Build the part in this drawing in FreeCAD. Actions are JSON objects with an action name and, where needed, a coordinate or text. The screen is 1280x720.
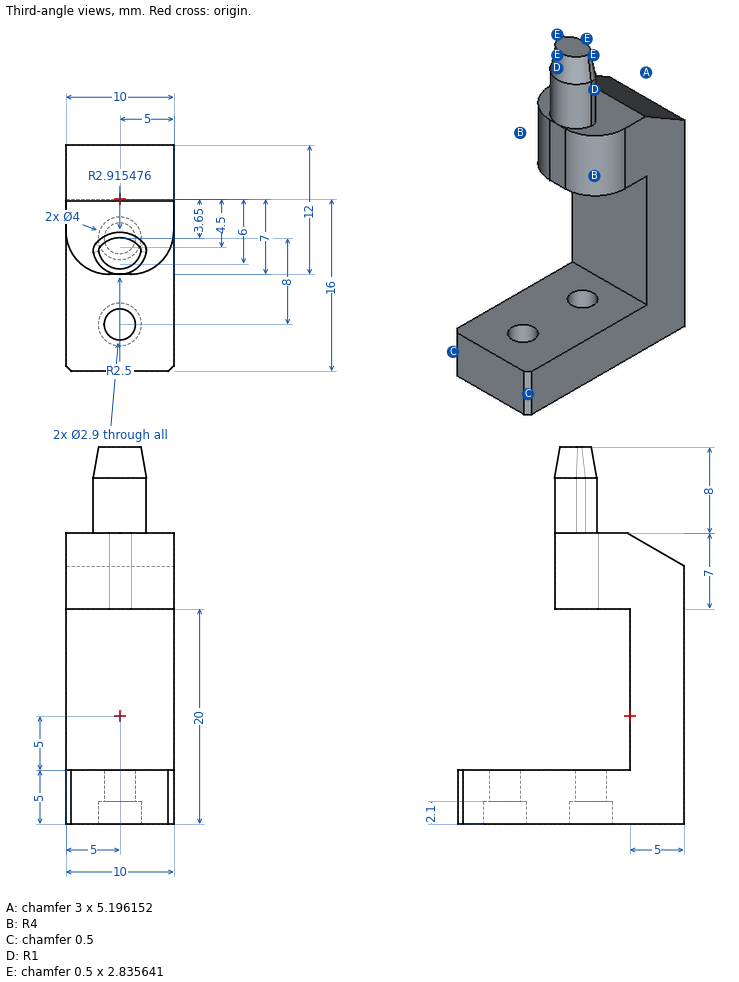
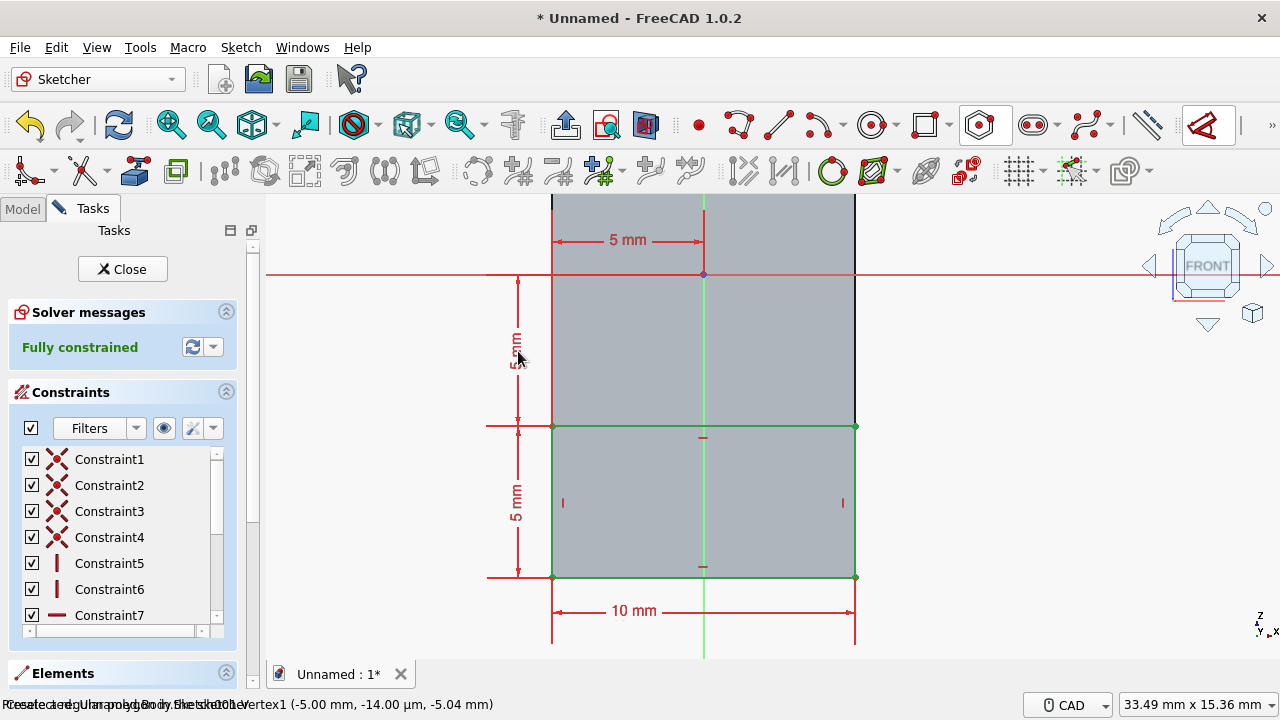
{"action": "left_click", "coordinate": [123, 269]}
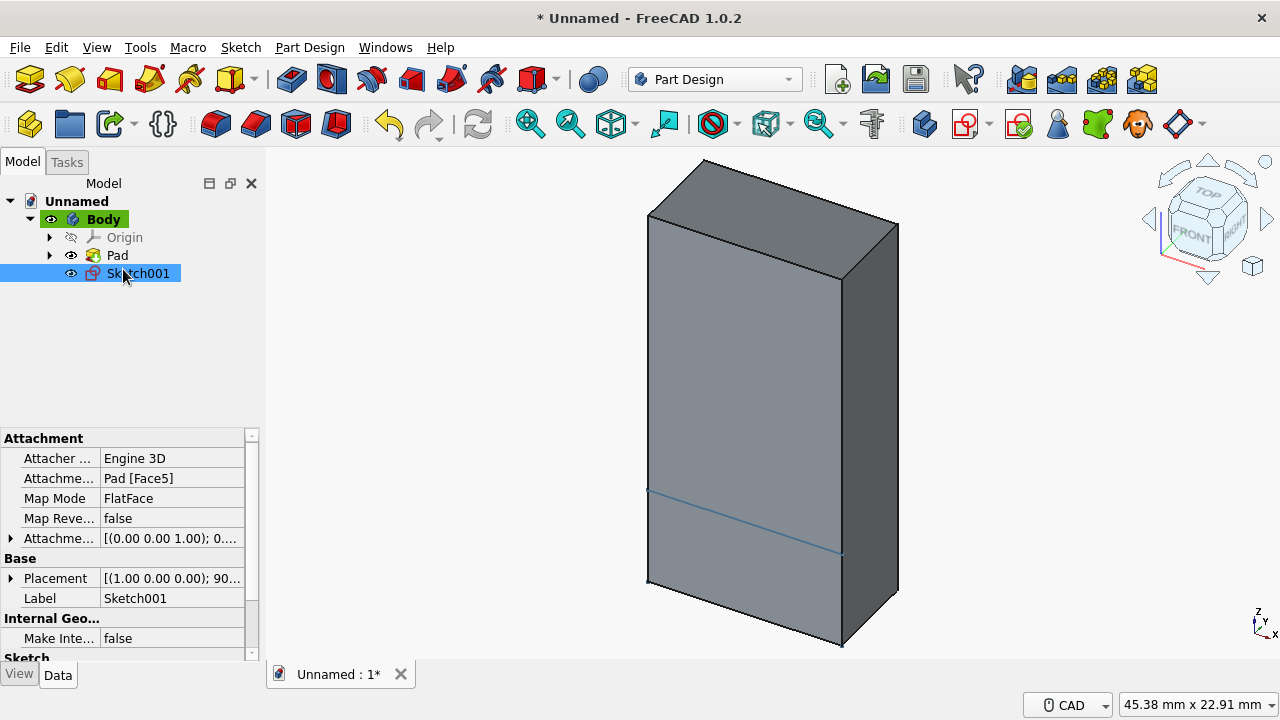
{"action": "left_click", "coordinate": [30, 80]}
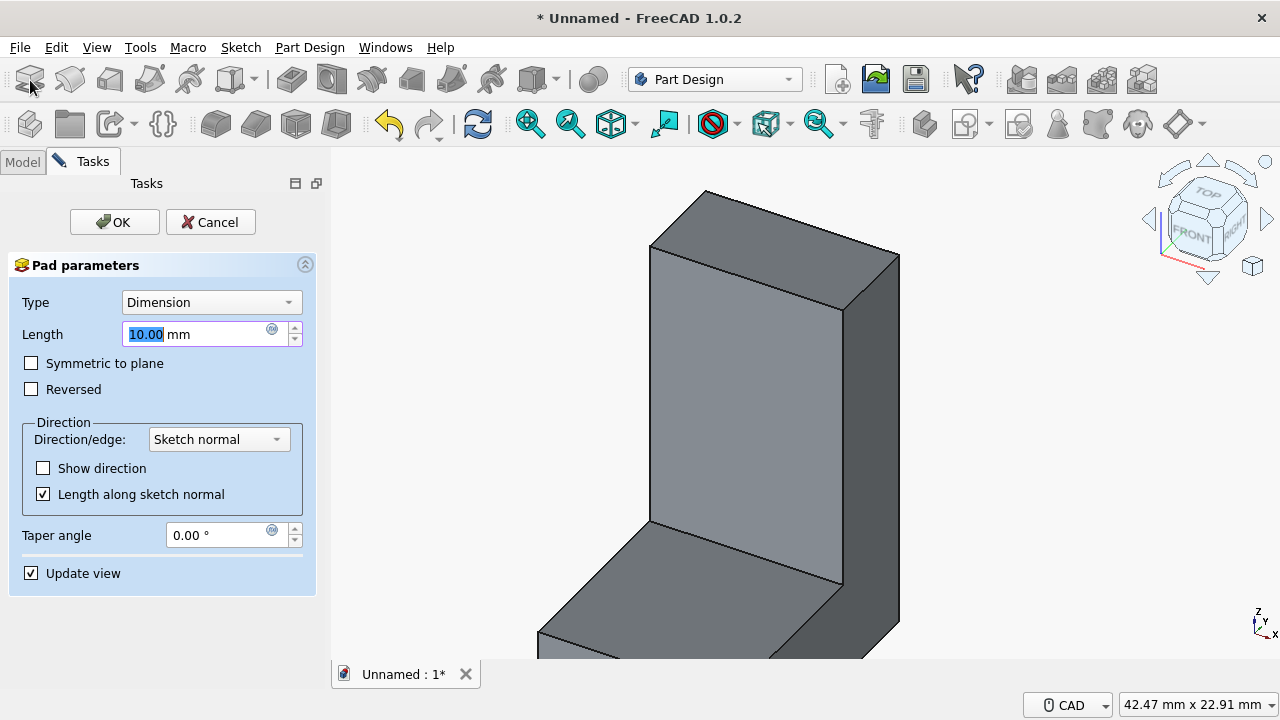
{"action": "type", "text": "16"}
{"action": "key", "text": "Tab"}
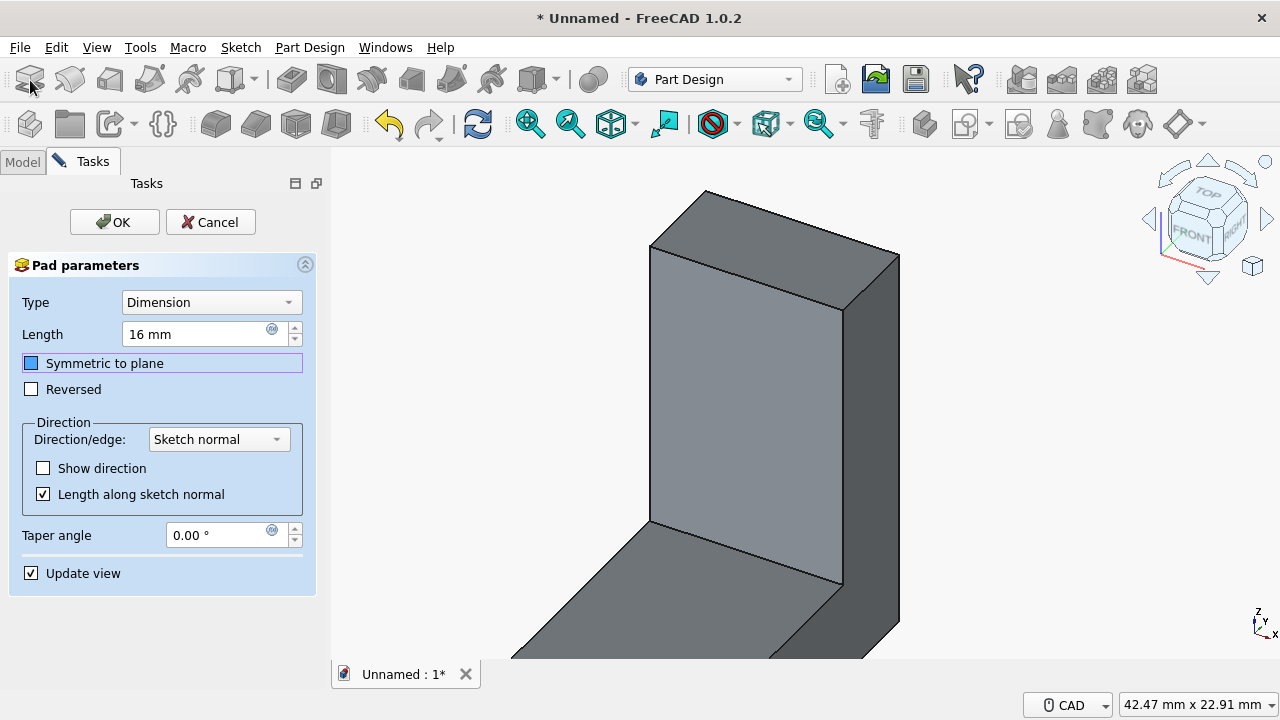
{"action": "left_click", "coordinate": [115, 222]}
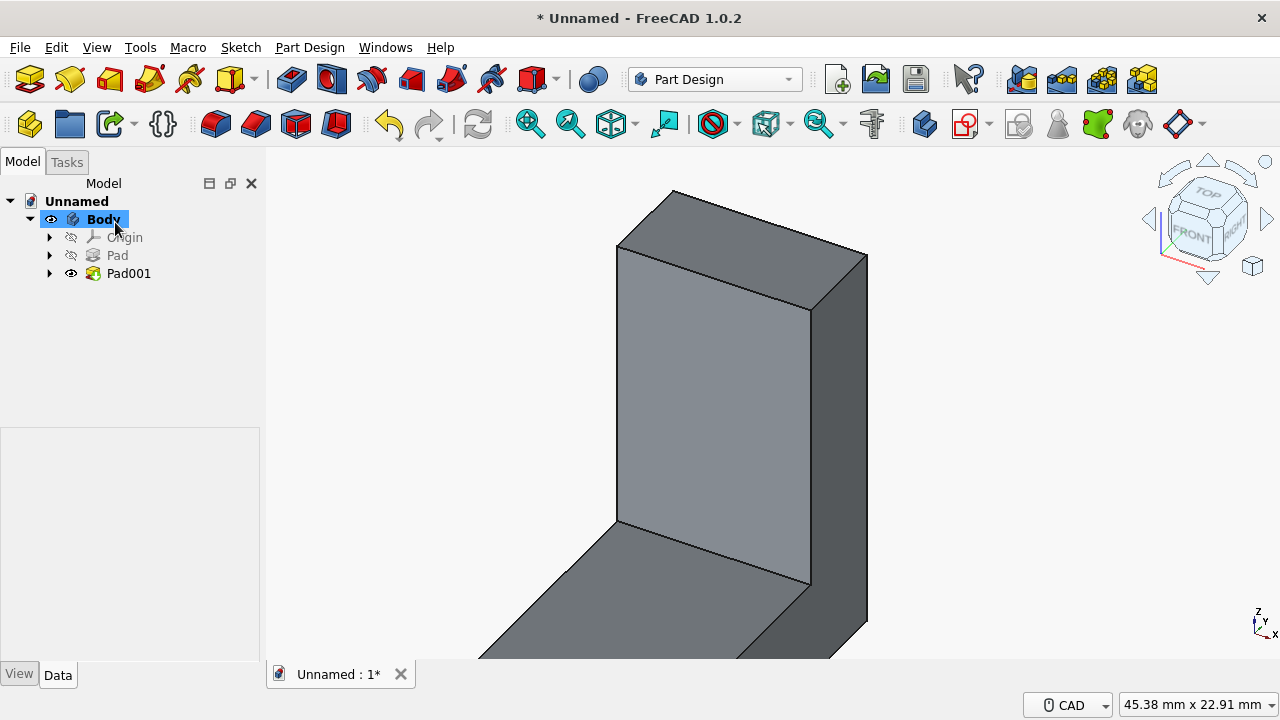
{"action": "left_click", "coordinate": [532, 124]}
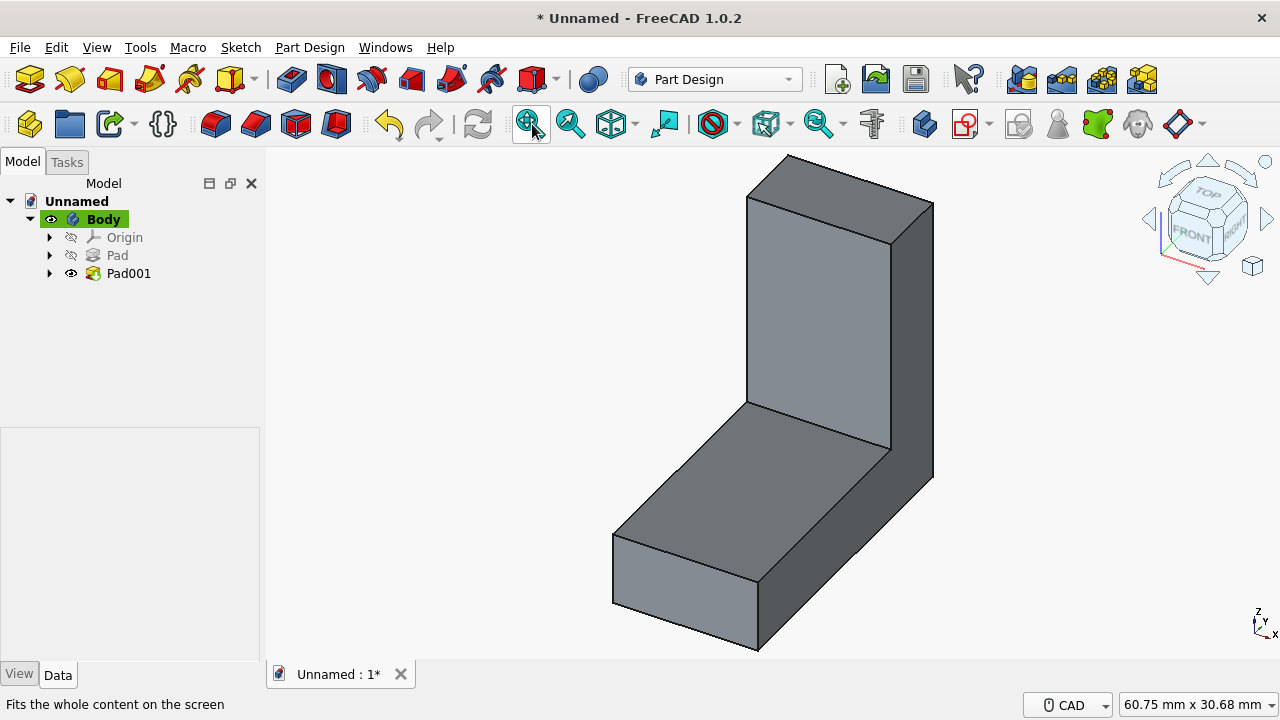
{"action": "left_click", "coordinate": [771, 472]}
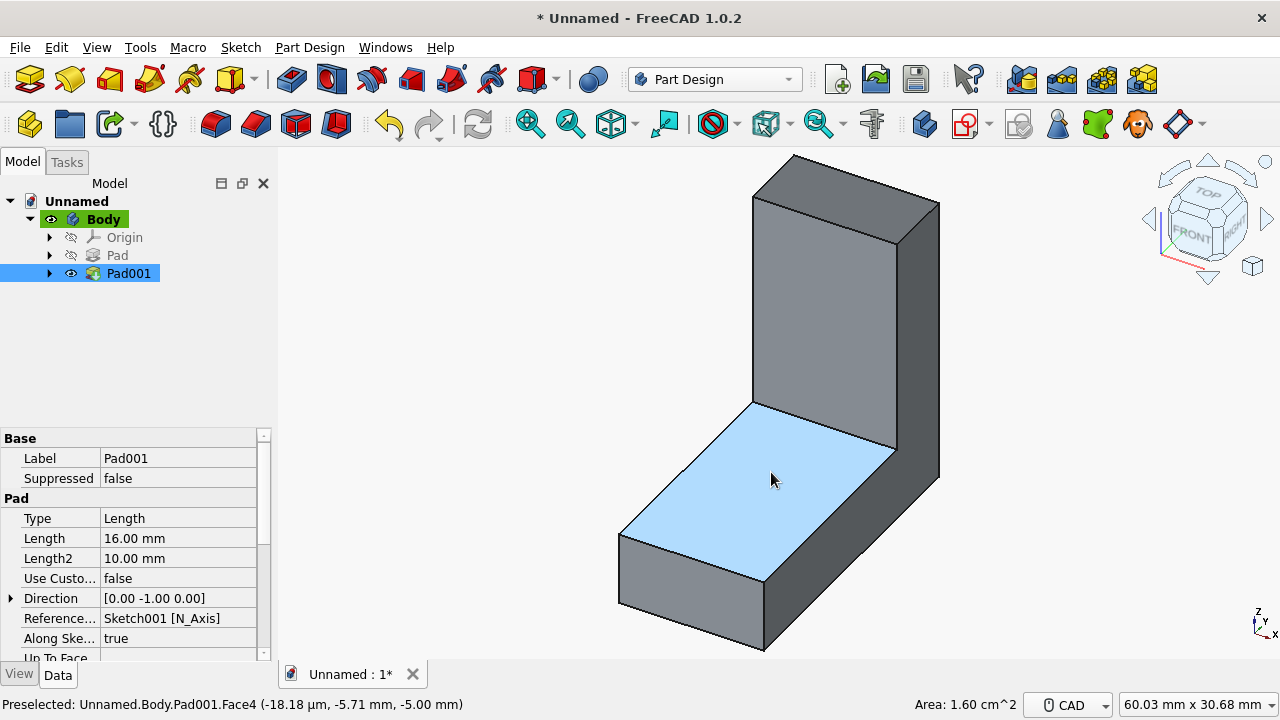
{"action": "left_click", "coordinate": [966, 124]}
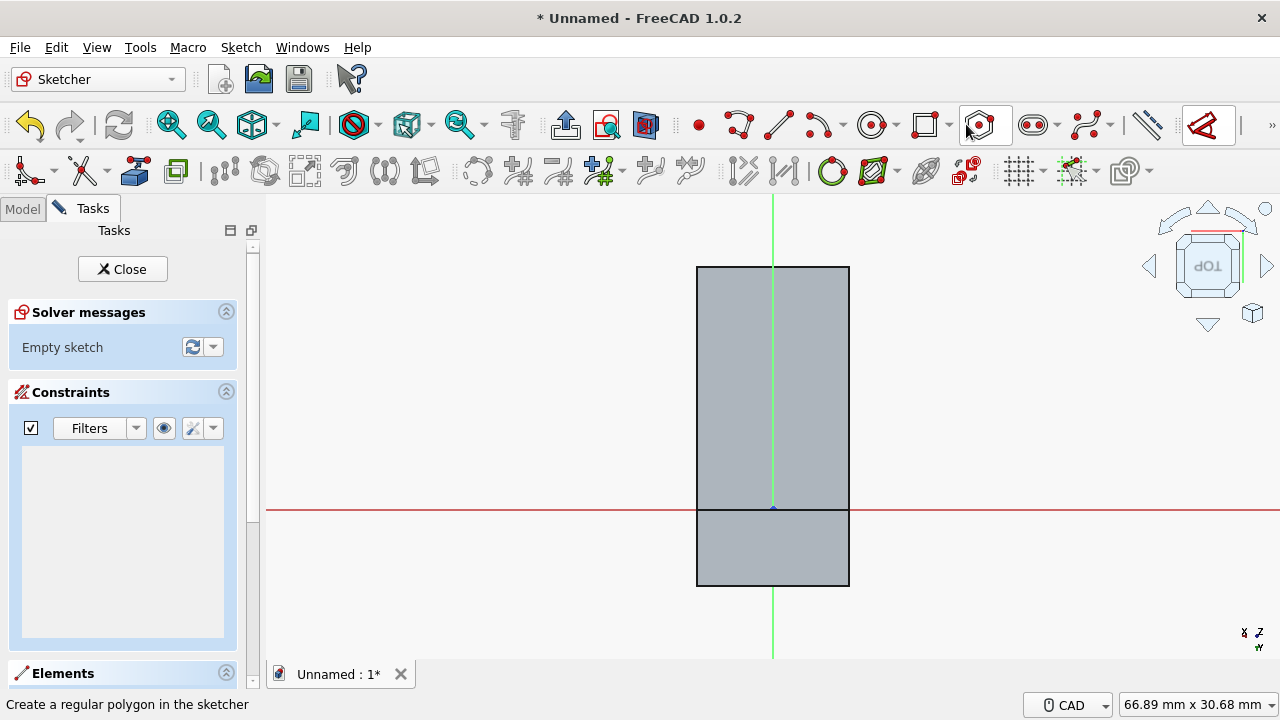
{"action": "scroll", "coordinate": [912, 378], "scroll_direction": "up", "scroll_amount": 2}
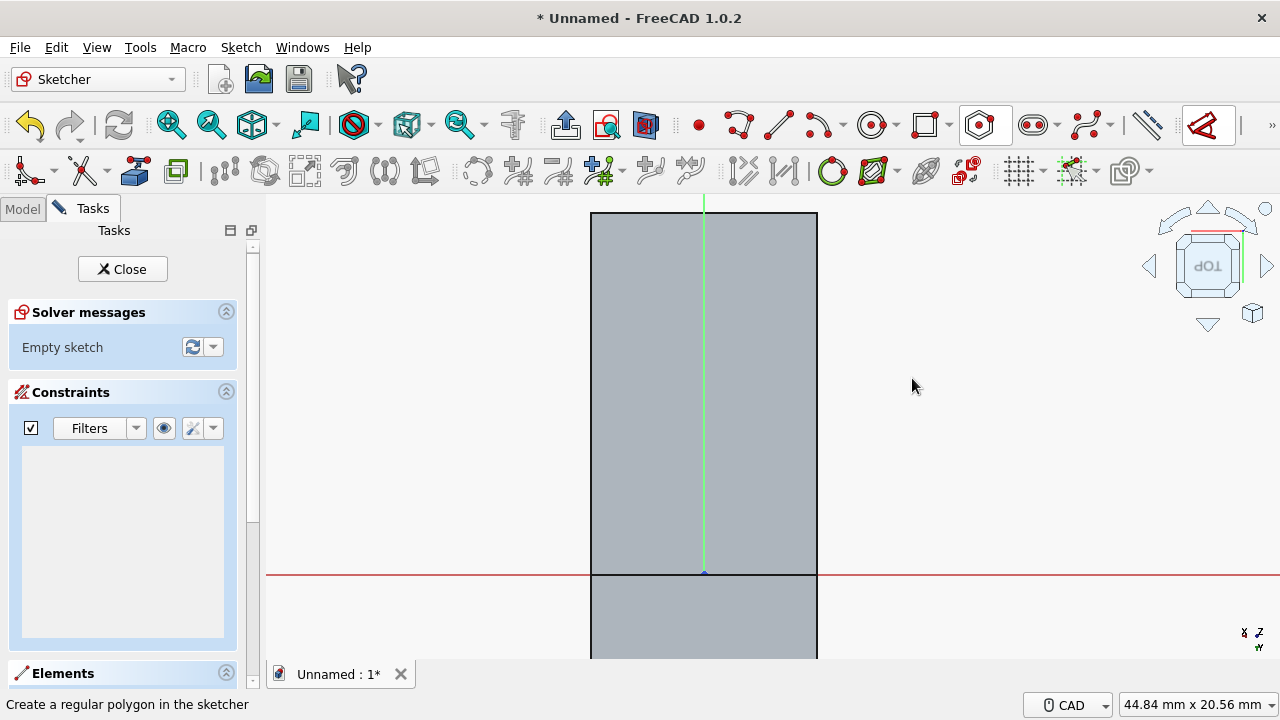
{"action": "key", "text": "g c"}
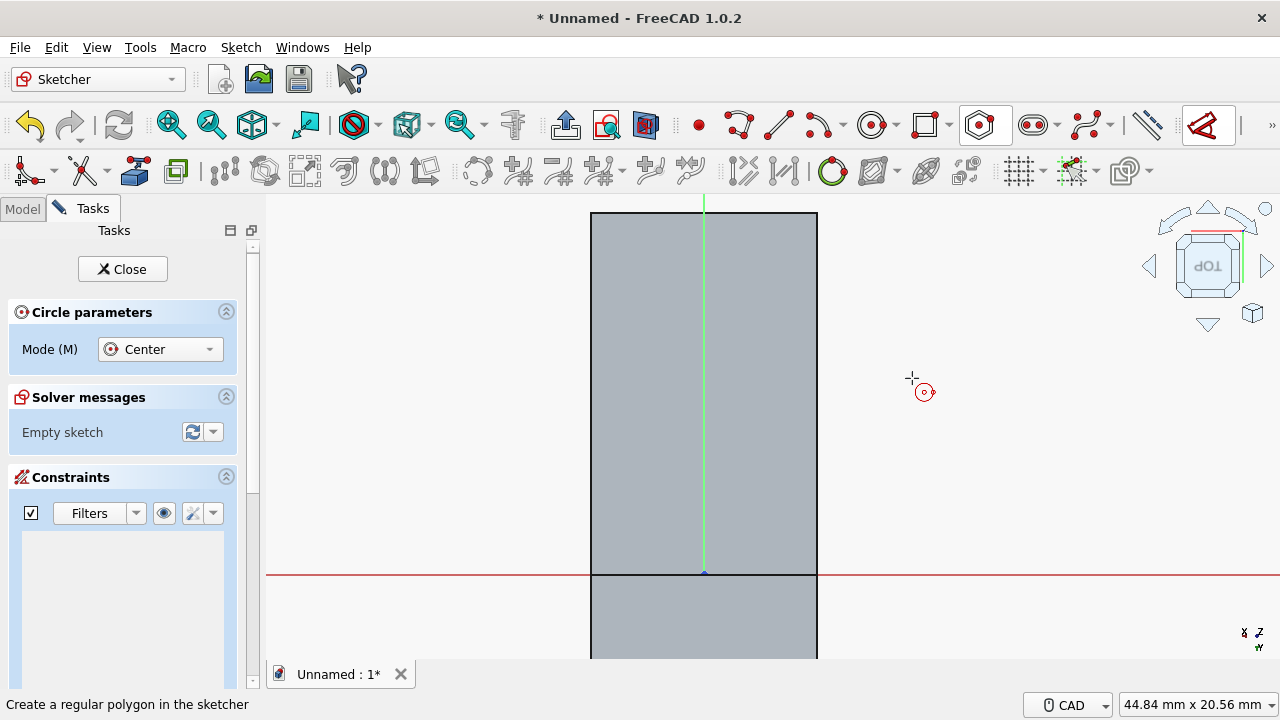
{"action": "left_click", "coordinate": [704, 311]}
{"action": "left_click", "coordinate": [728, 288]}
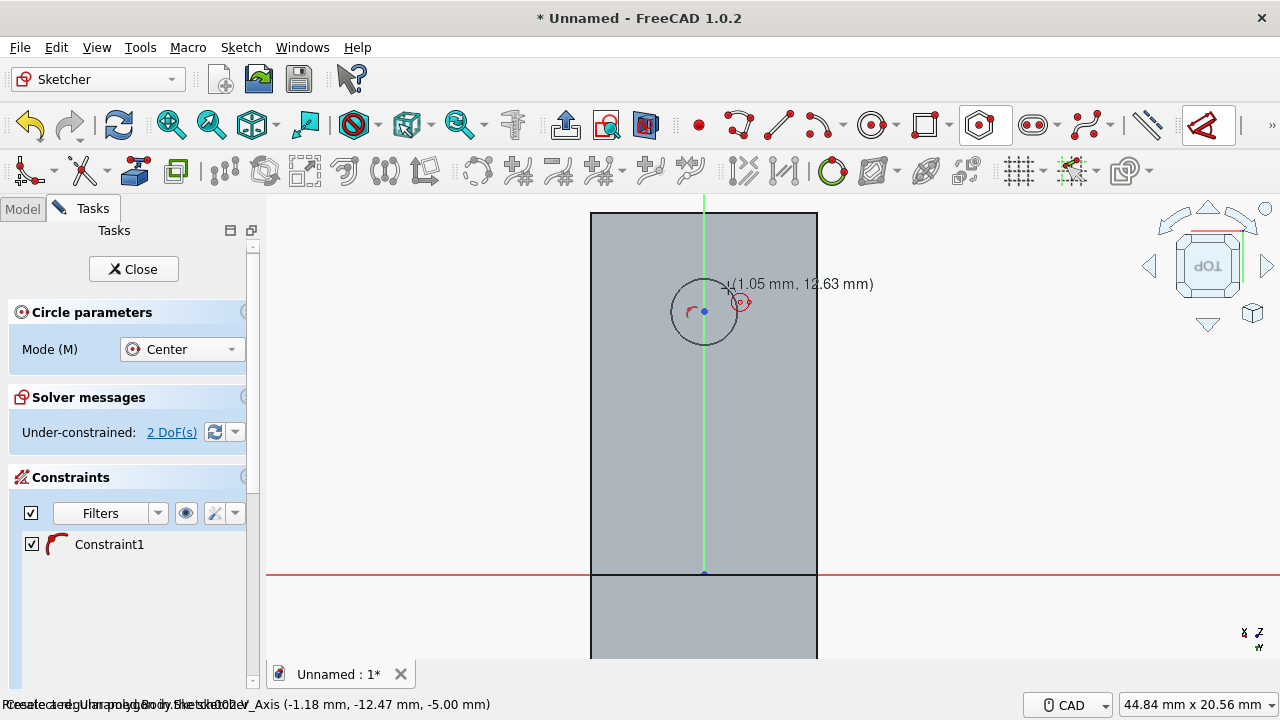
{"action": "left_click", "coordinate": [704, 492]}
{"action": "left_click", "coordinate": [728, 469]}
{"action": "key", "text": "Escape"}